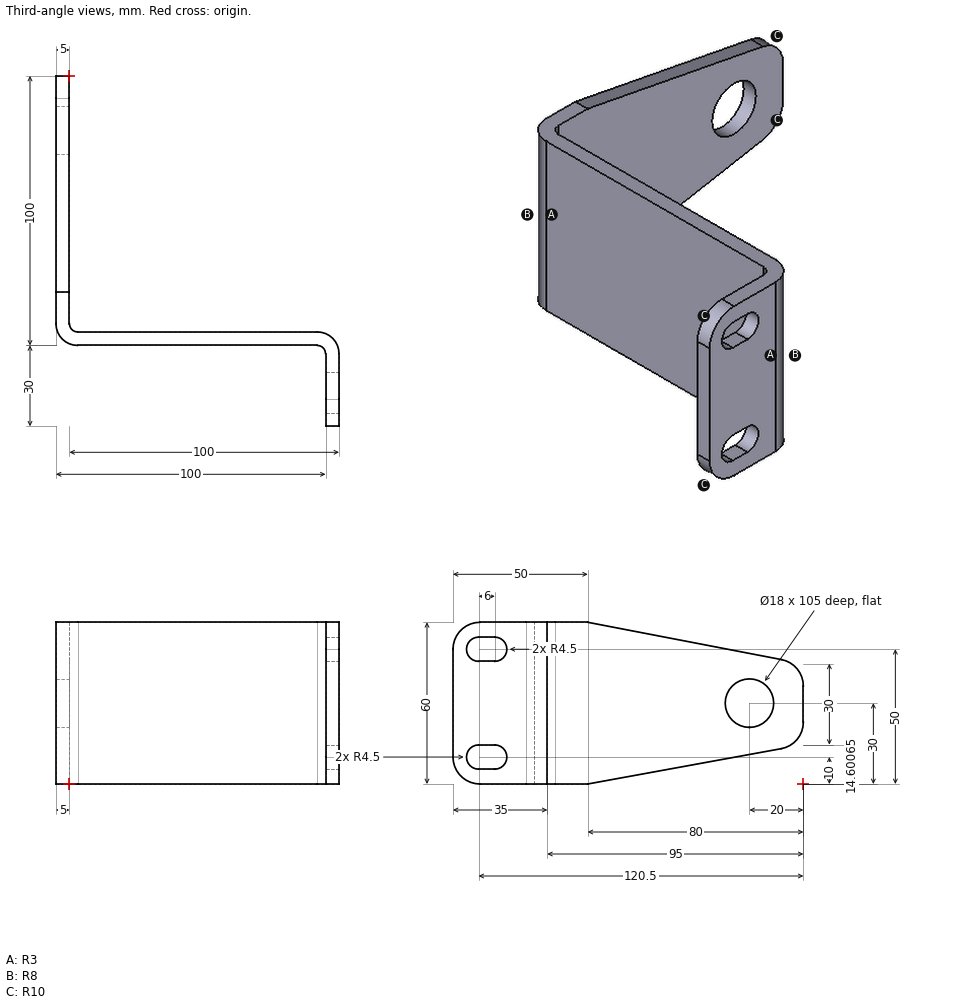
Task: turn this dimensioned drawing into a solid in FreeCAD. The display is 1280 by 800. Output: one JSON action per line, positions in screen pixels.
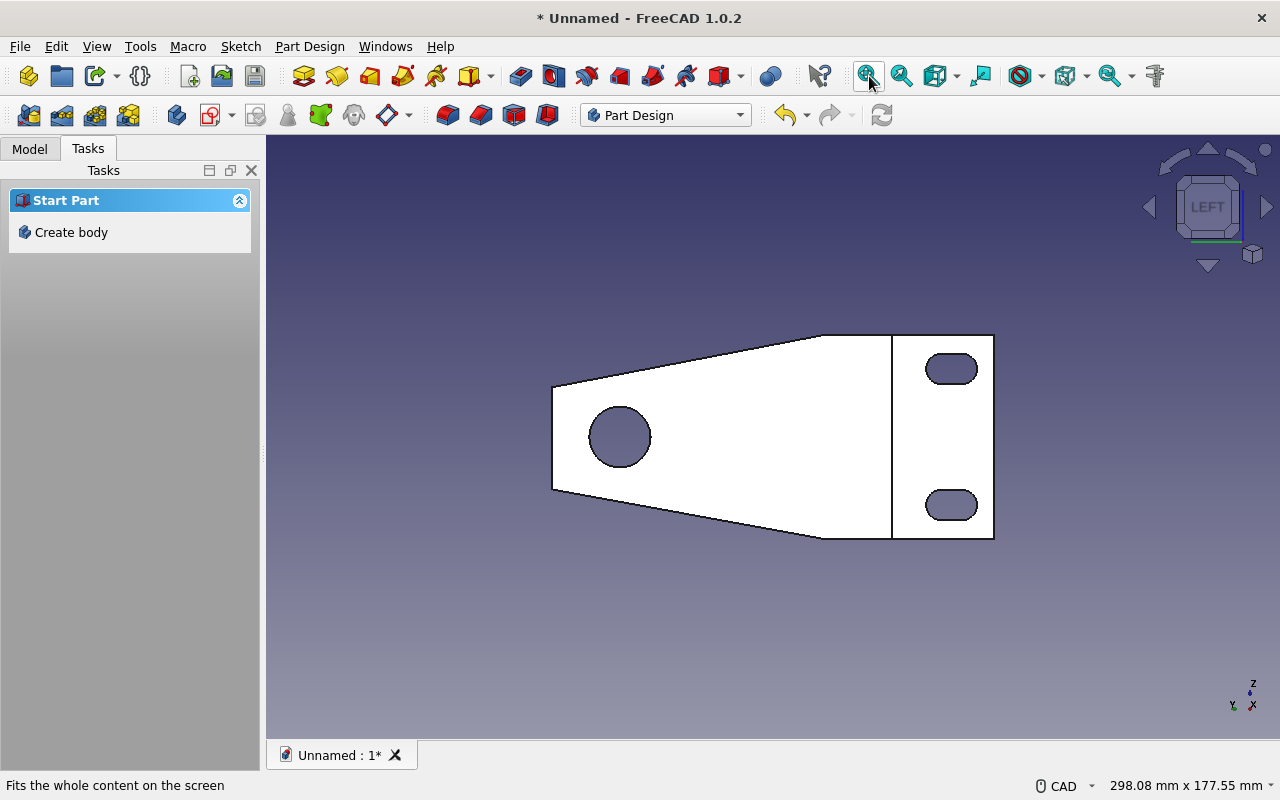
{"action": "key", "text": "v 3"}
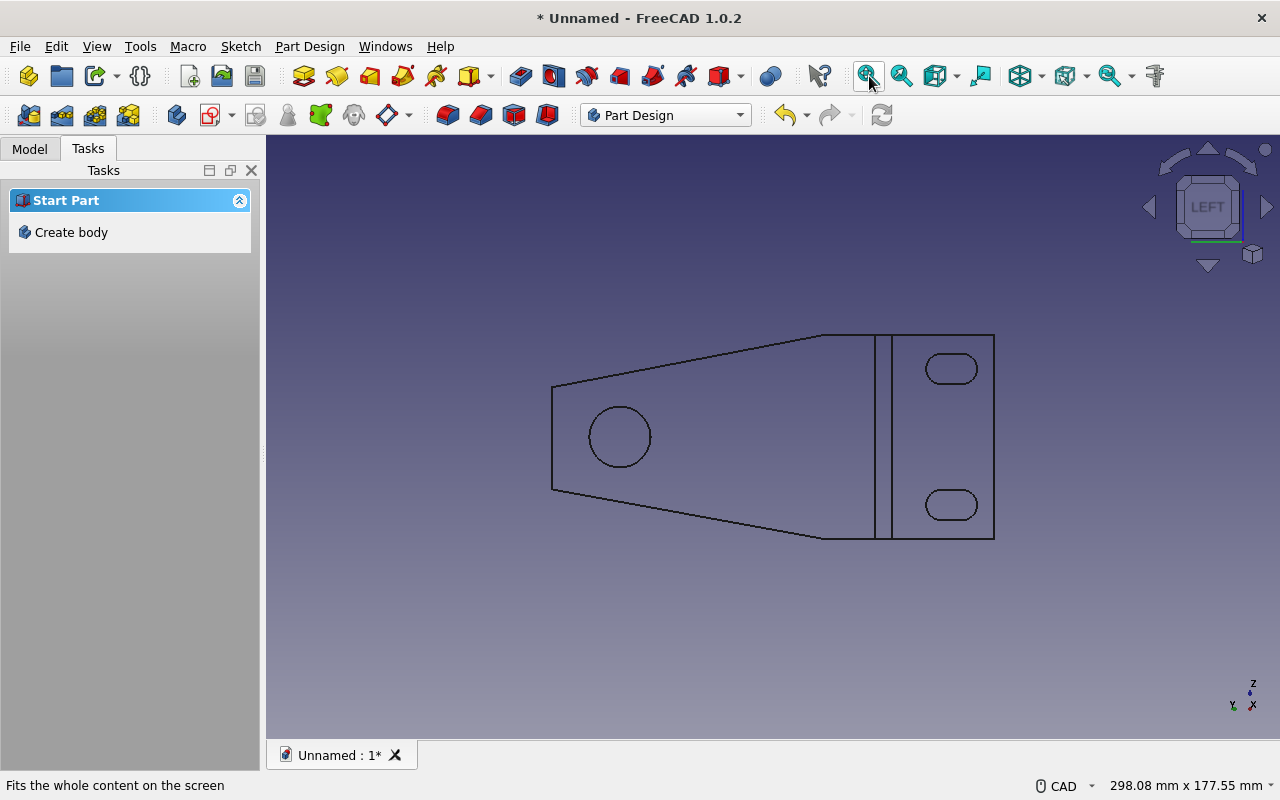
{"action": "key", "text": "0"}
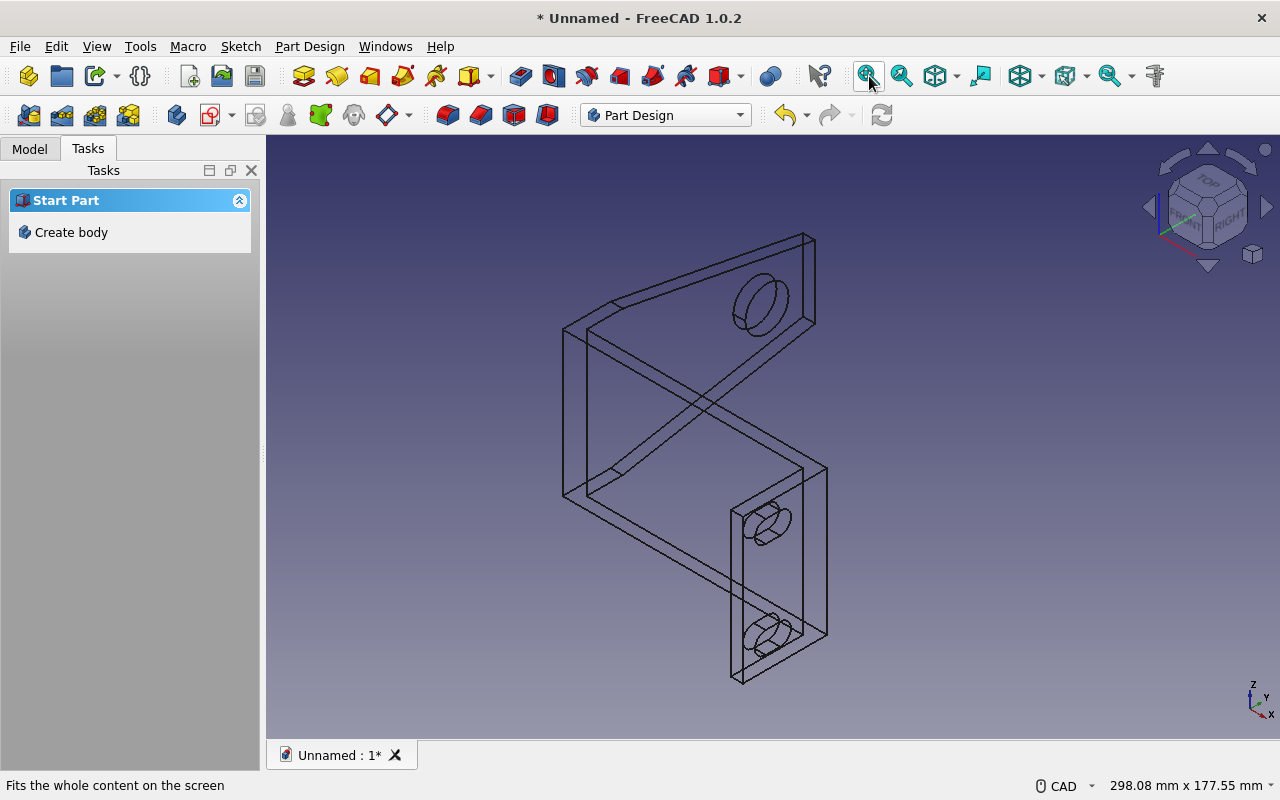
{"action": "left_click", "coordinate": [587, 412]}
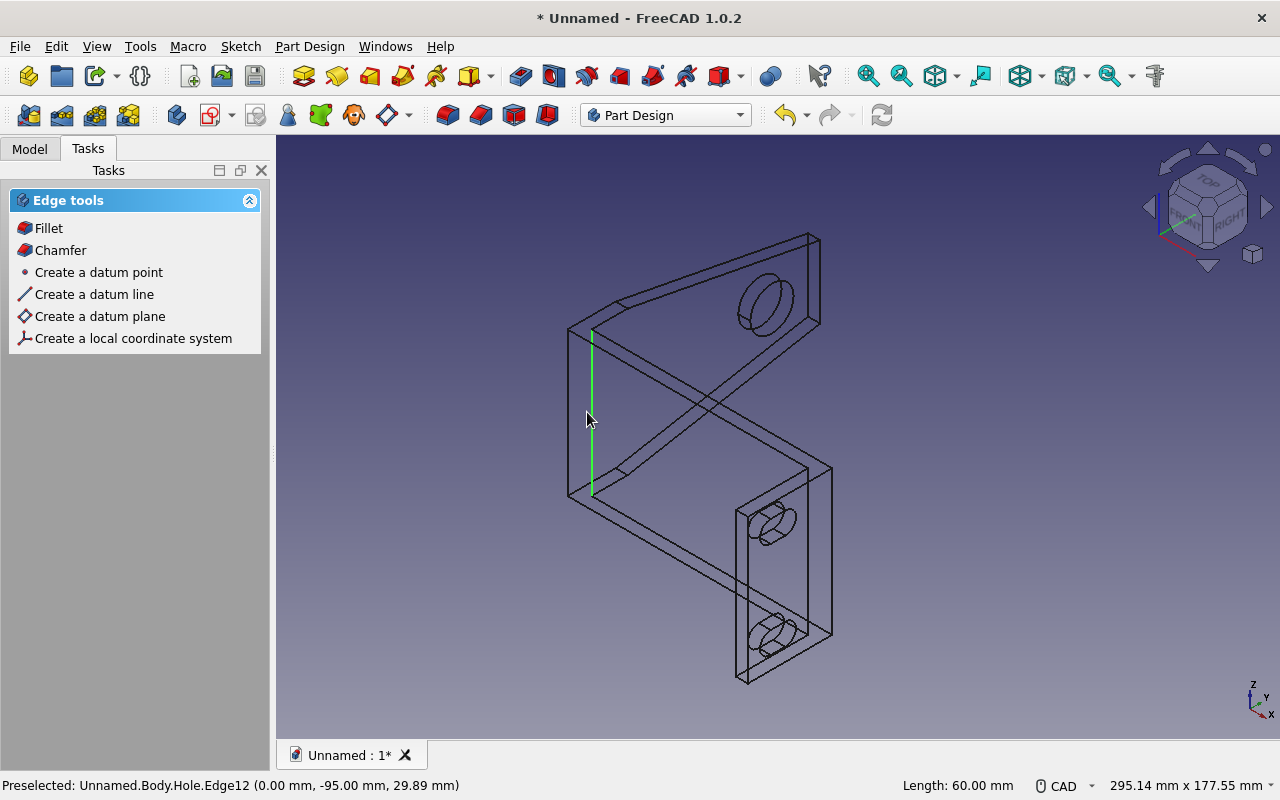
{"action": "left_click", "coordinate": [808, 551], "text": "ctrl"}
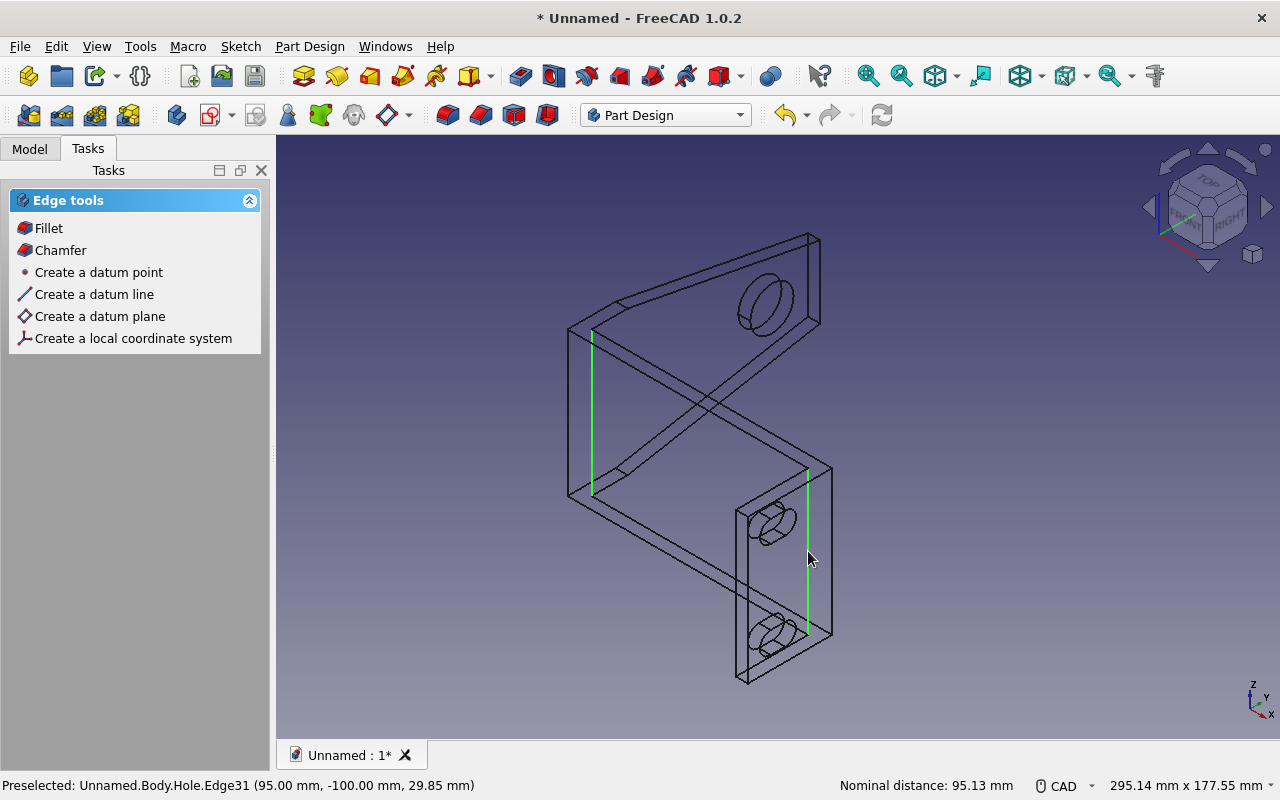
{"action": "key", "text": "v 1"}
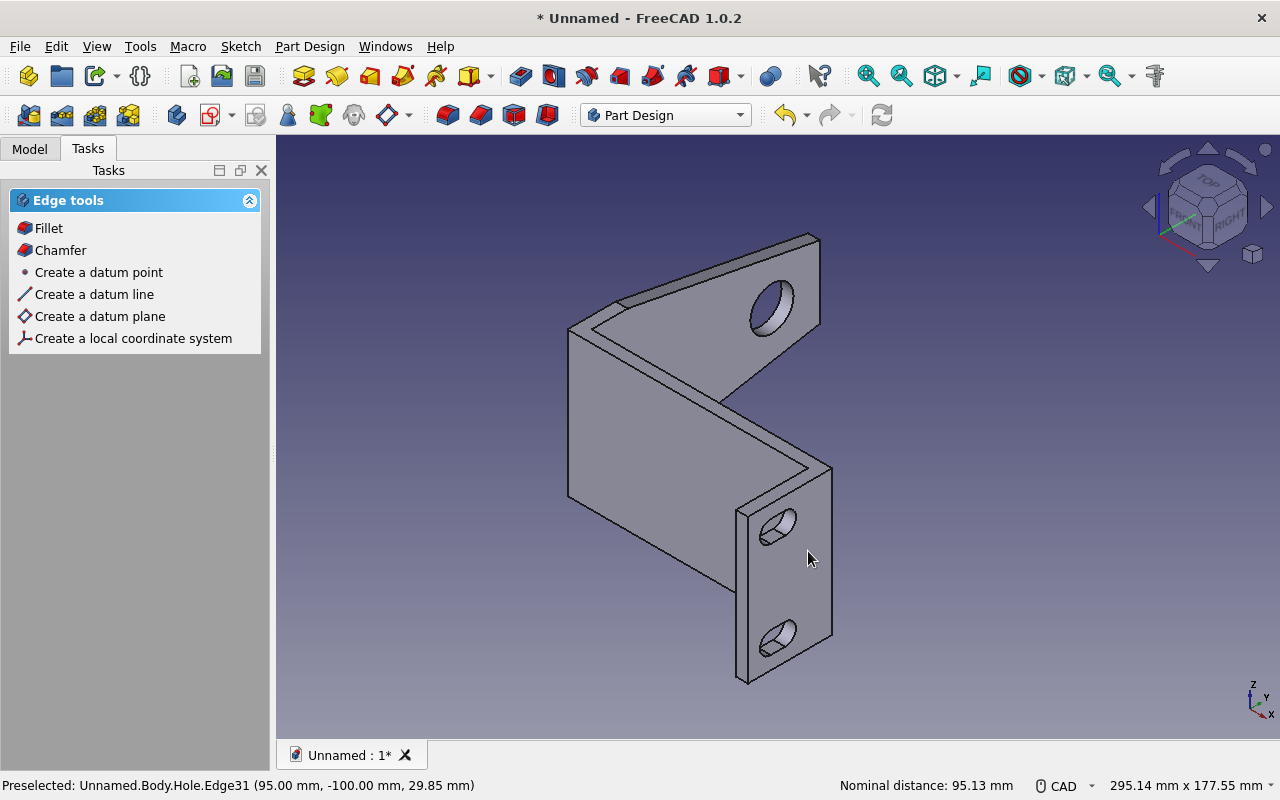
{"action": "left_click", "coordinate": [448, 116]}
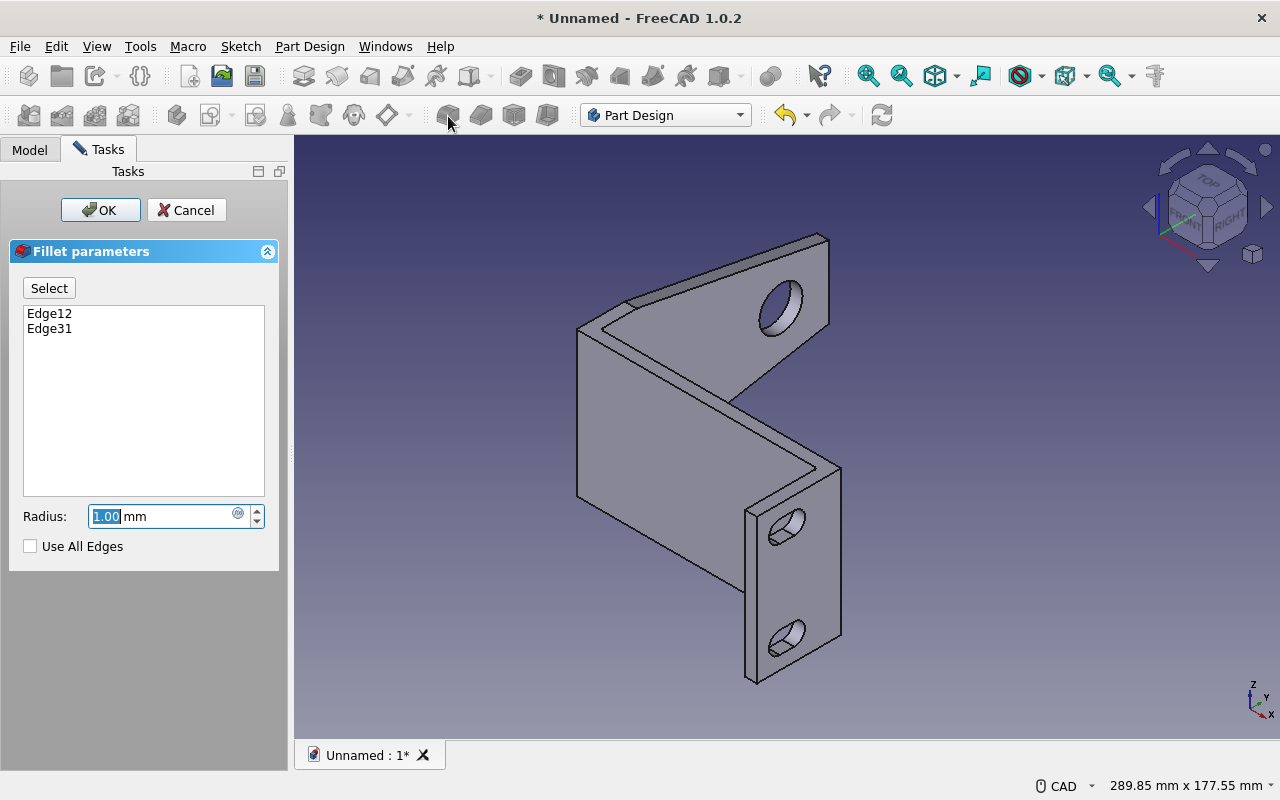
{"action": "type", "text": "3"}
{"action": "key", "text": "Tab"}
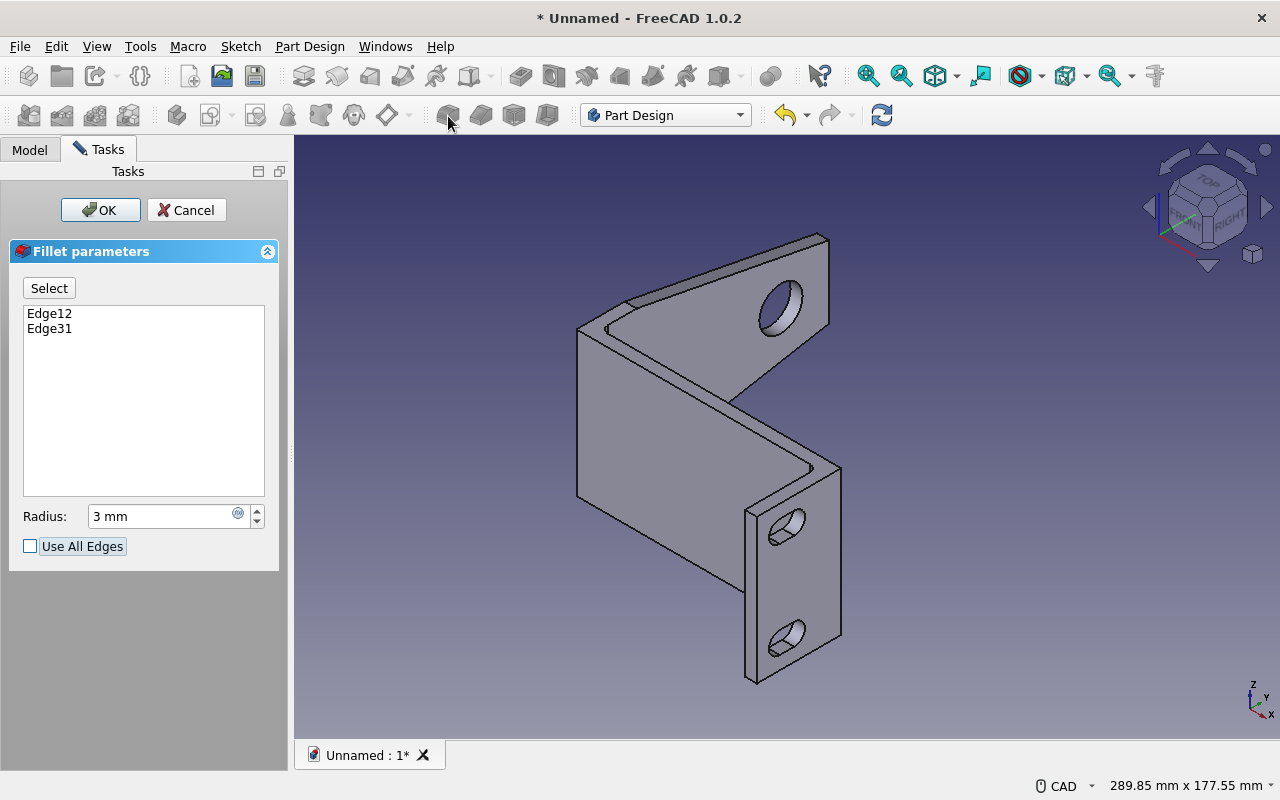
{"action": "left_click", "coordinate": [101, 210]}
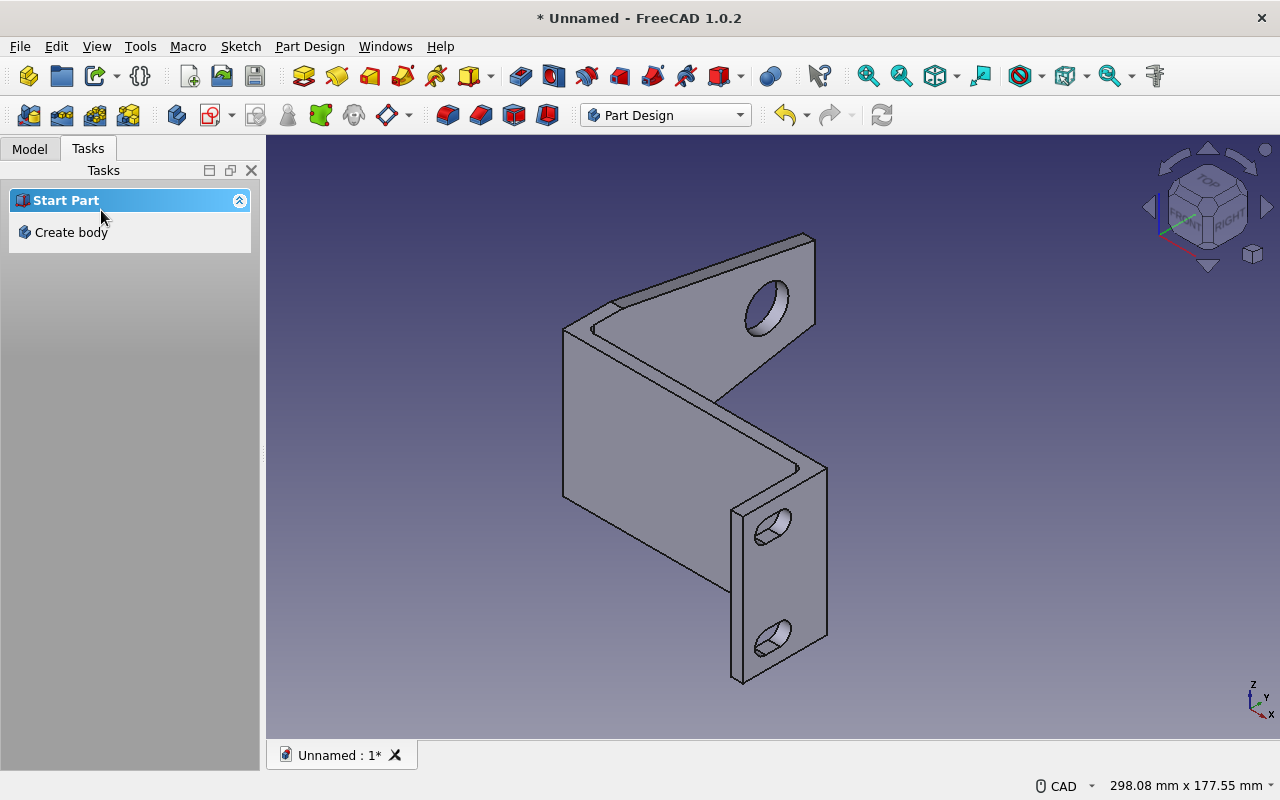
{"action": "key", "text": "2"}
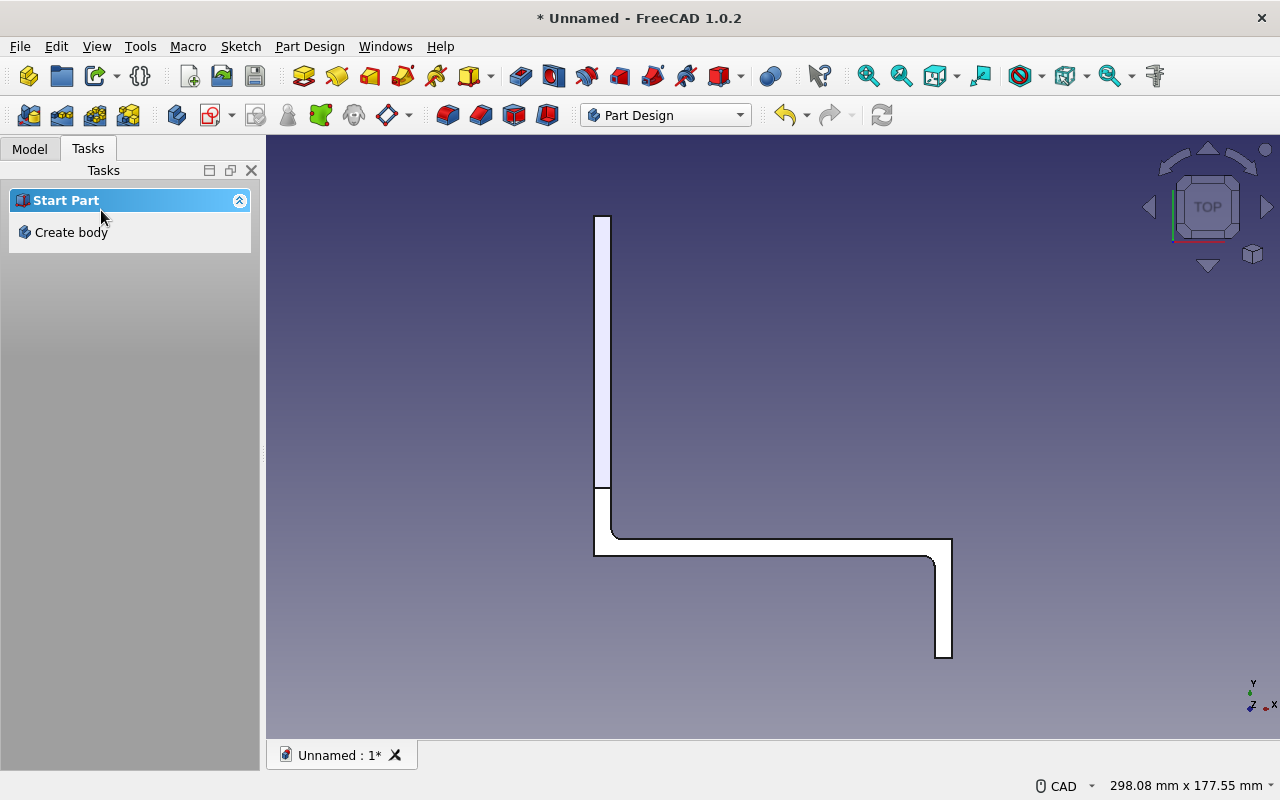
{"action": "key", "text": "0"}